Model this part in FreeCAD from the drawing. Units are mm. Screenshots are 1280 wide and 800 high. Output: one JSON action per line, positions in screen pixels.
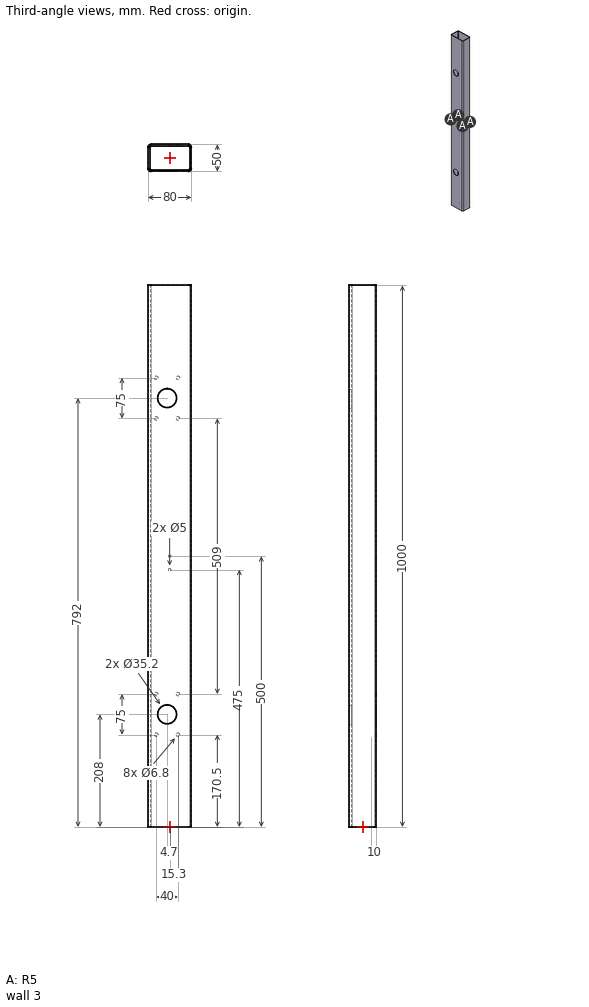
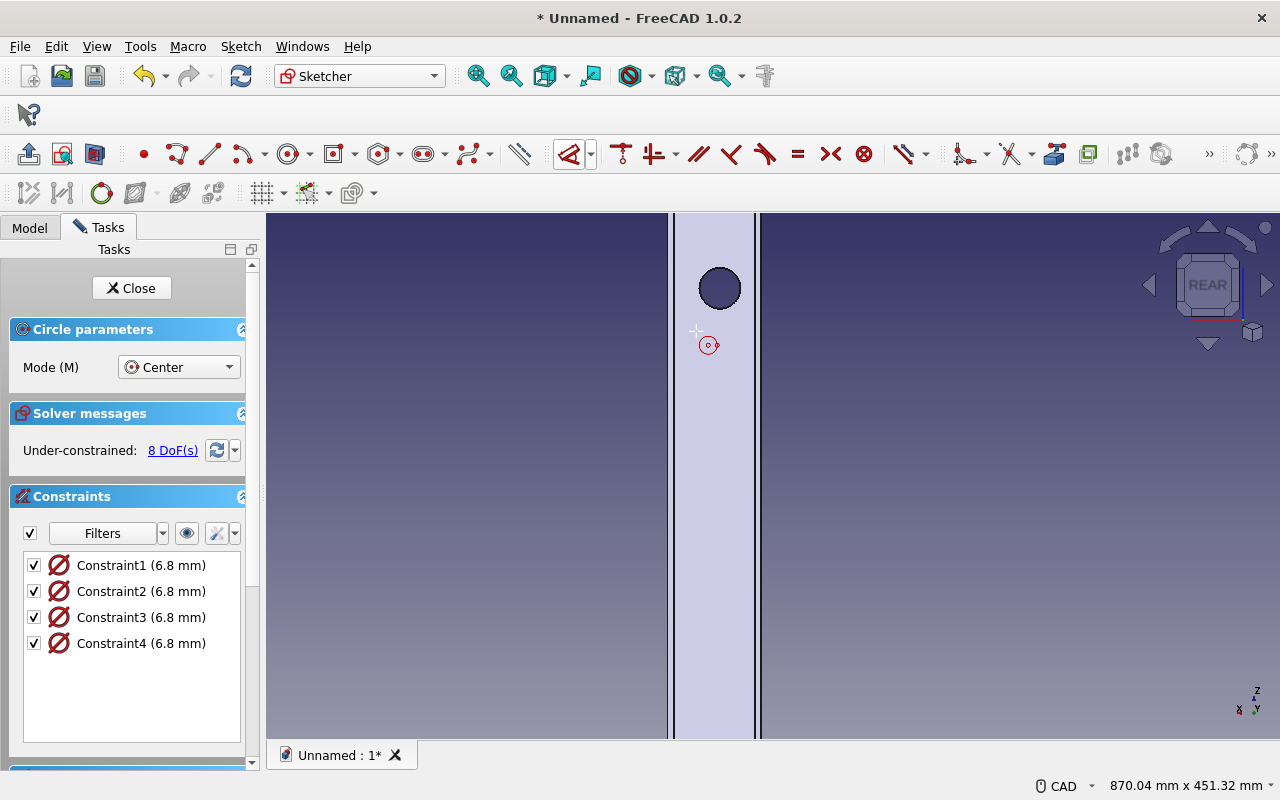
{"action": "left_click", "coordinate": [697, 332]}
{"action": "mouse_move", "coordinate": [699, 329]}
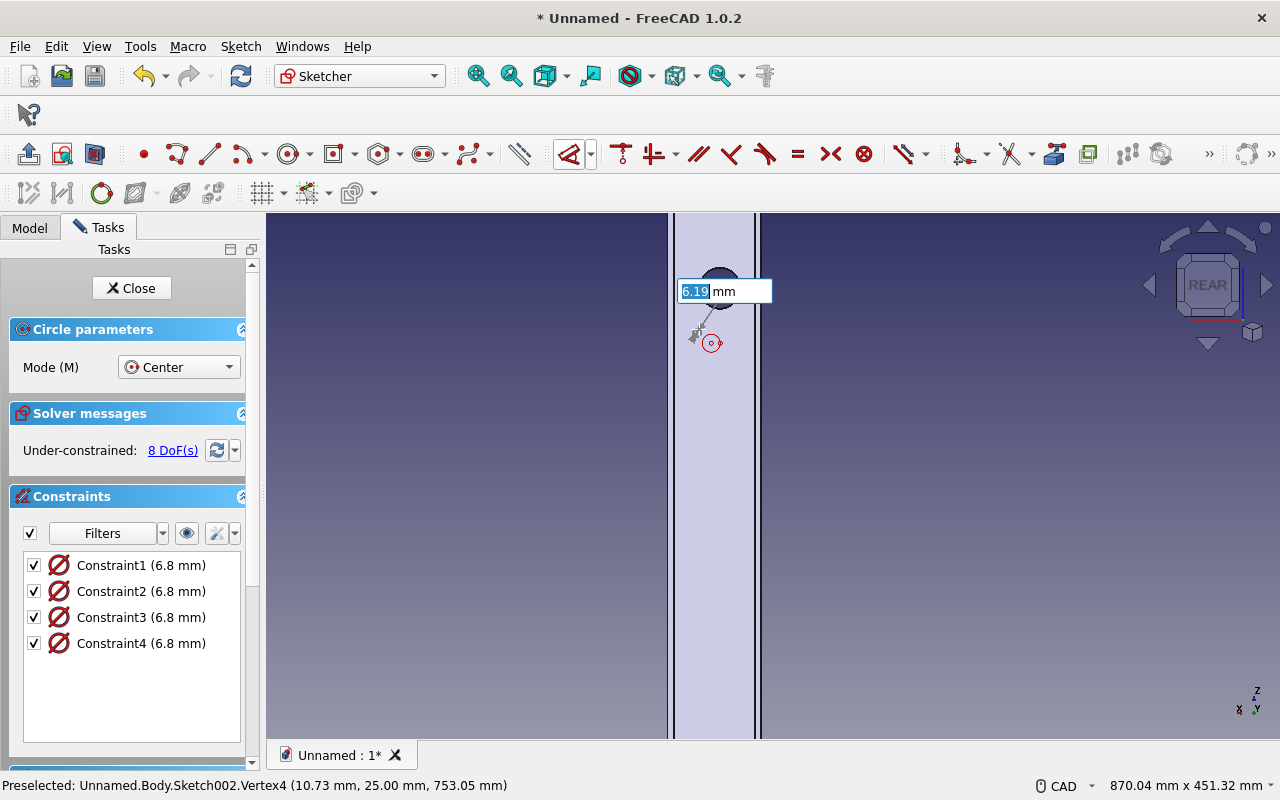
{"action": "type", "text": "6.8"}
{"action": "key", "text": "Return"}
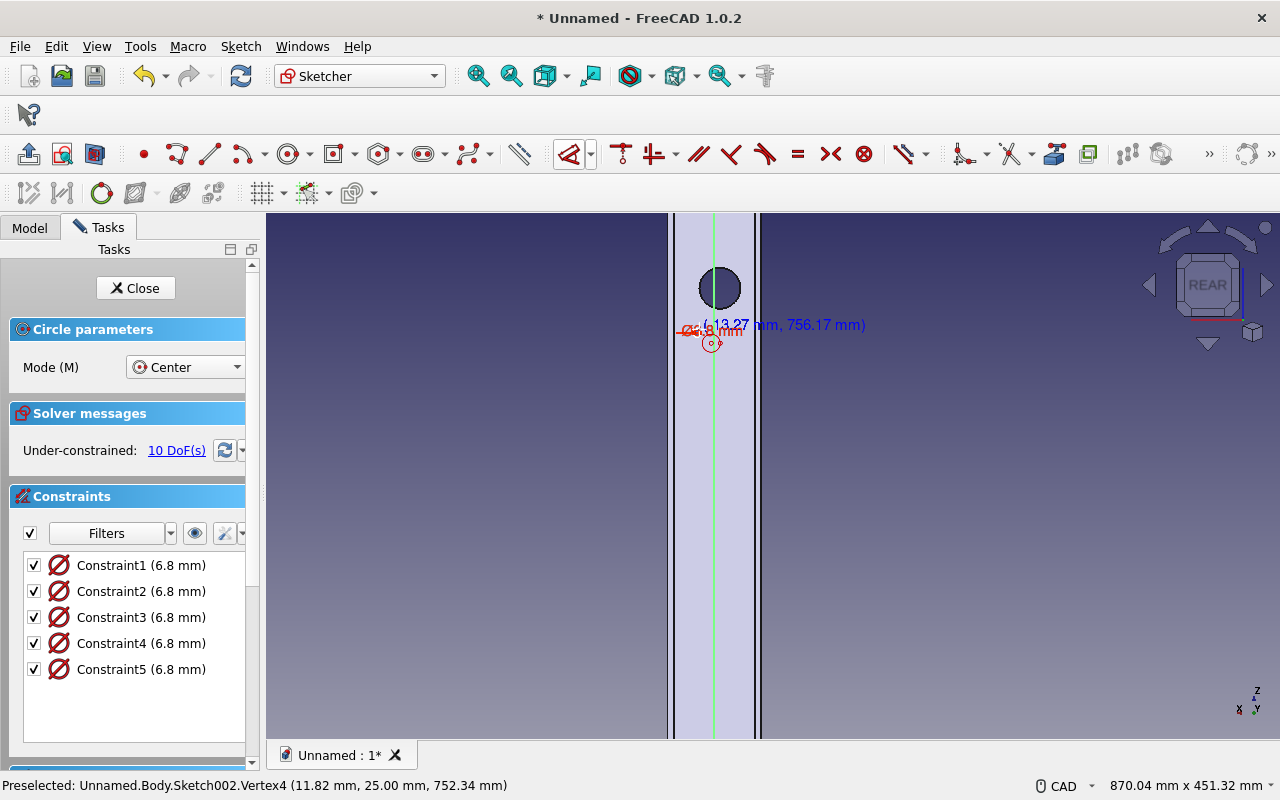
{"action": "scroll", "coordinate": [743, 332], "scroll_direction": "up", "scroll_amount": 9}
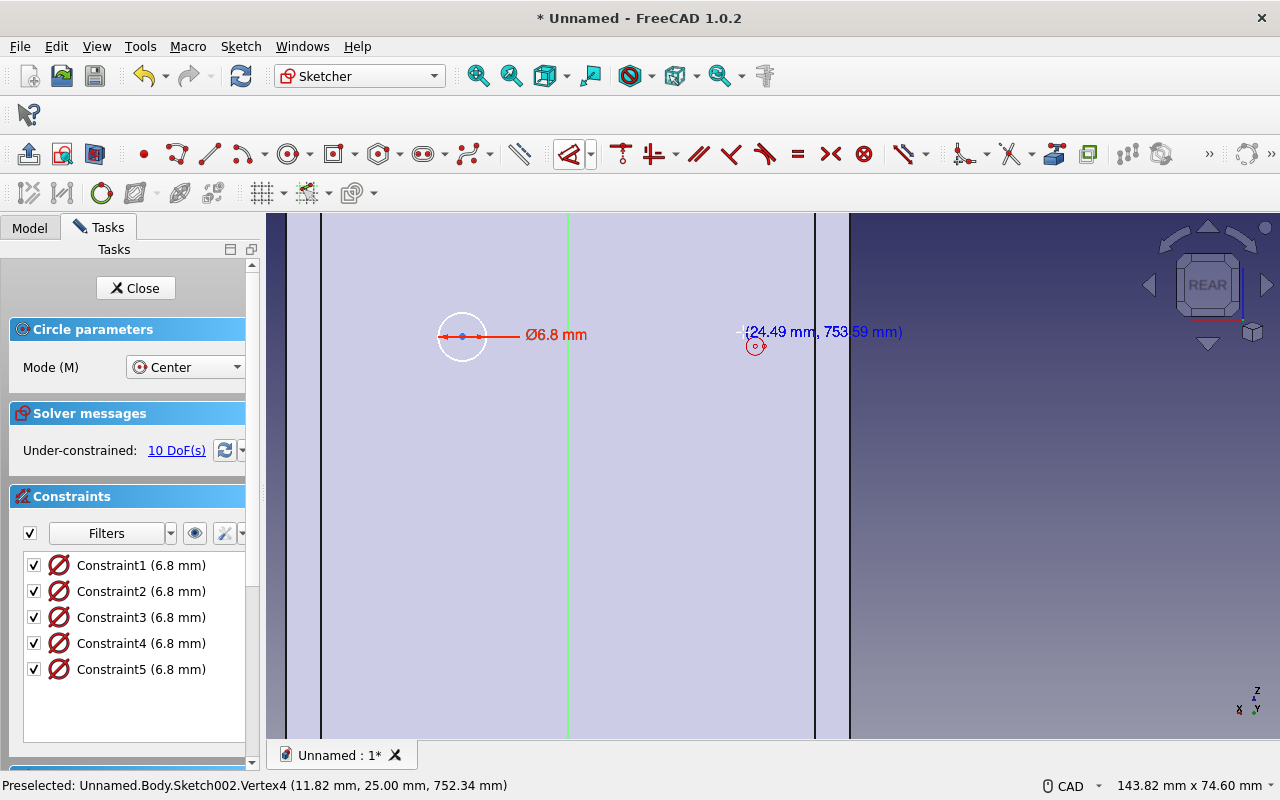
{"action": "scroll", "coordinate": [711, 331], "scroll_direction": "down", "scroll_amount": 14}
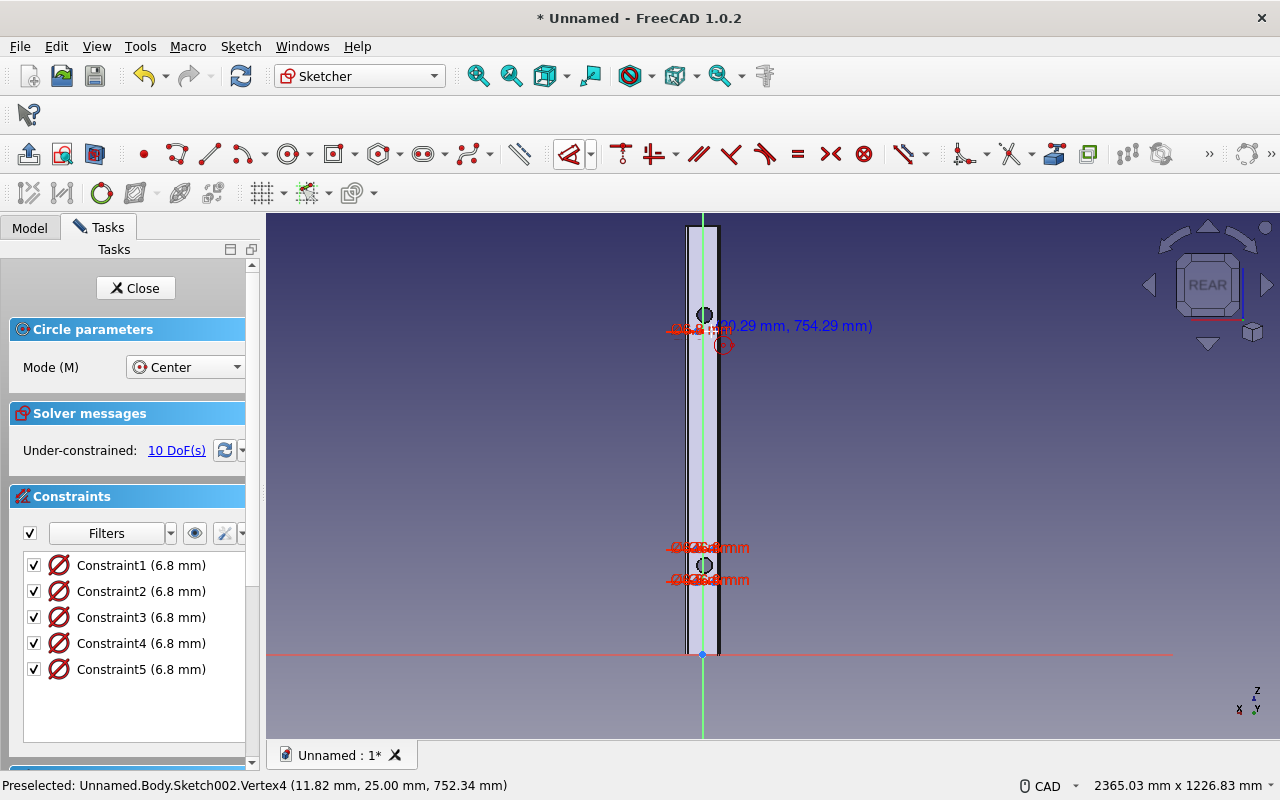
{"action": "scroll", "coordinate": [713, 331], "scroll_direction": "up", "scroll_amount": 3}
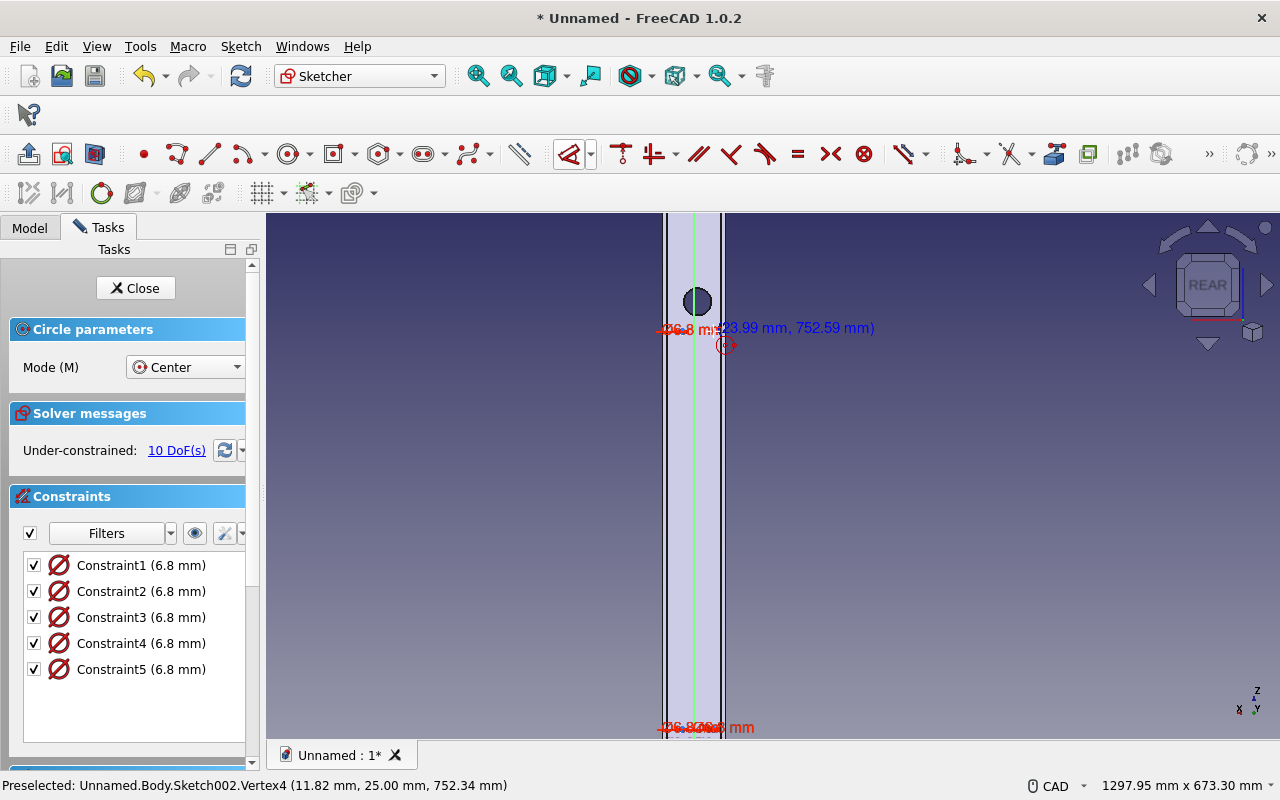
{"action": "left_click", "coordinate": [713, 331]}
{"action": "mouse_move", "coordinate": [715, 329]}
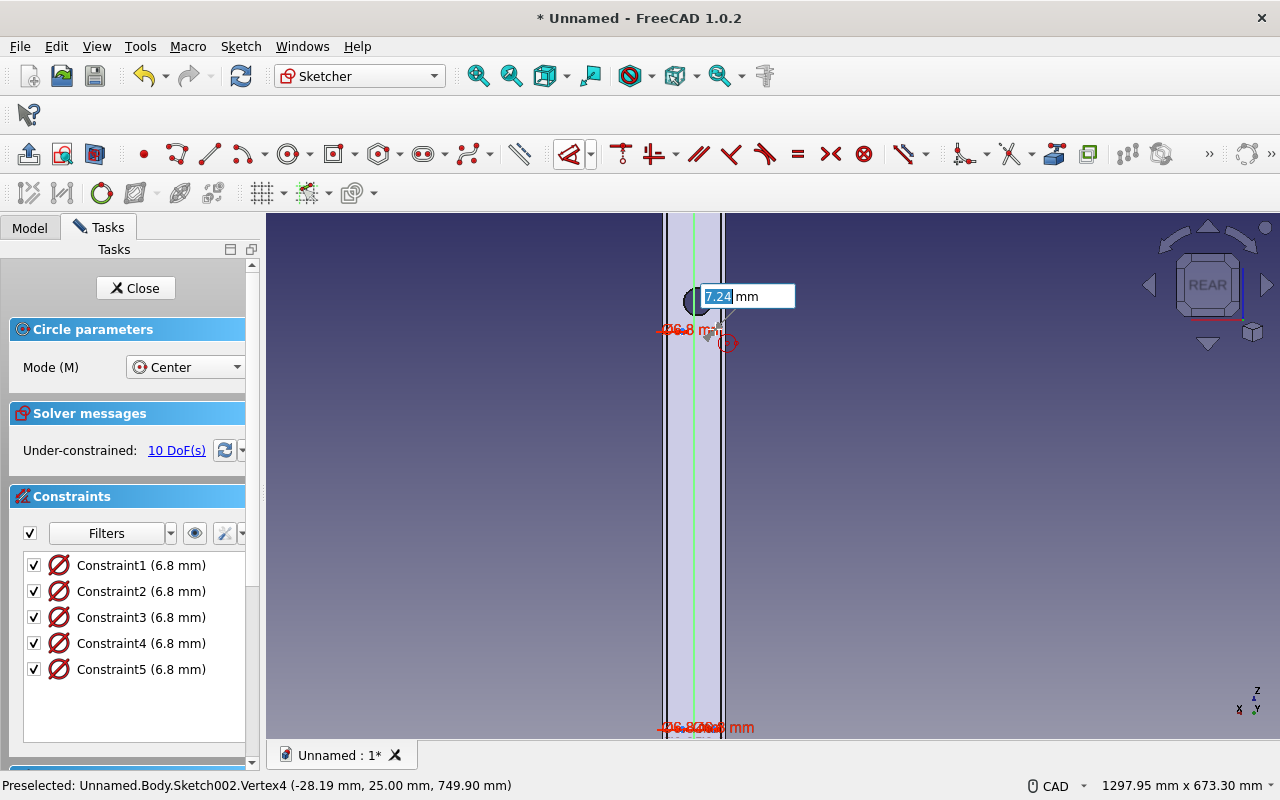
{"action": "type", "text": "6.8"}
{"action": "key", "text": "Return"}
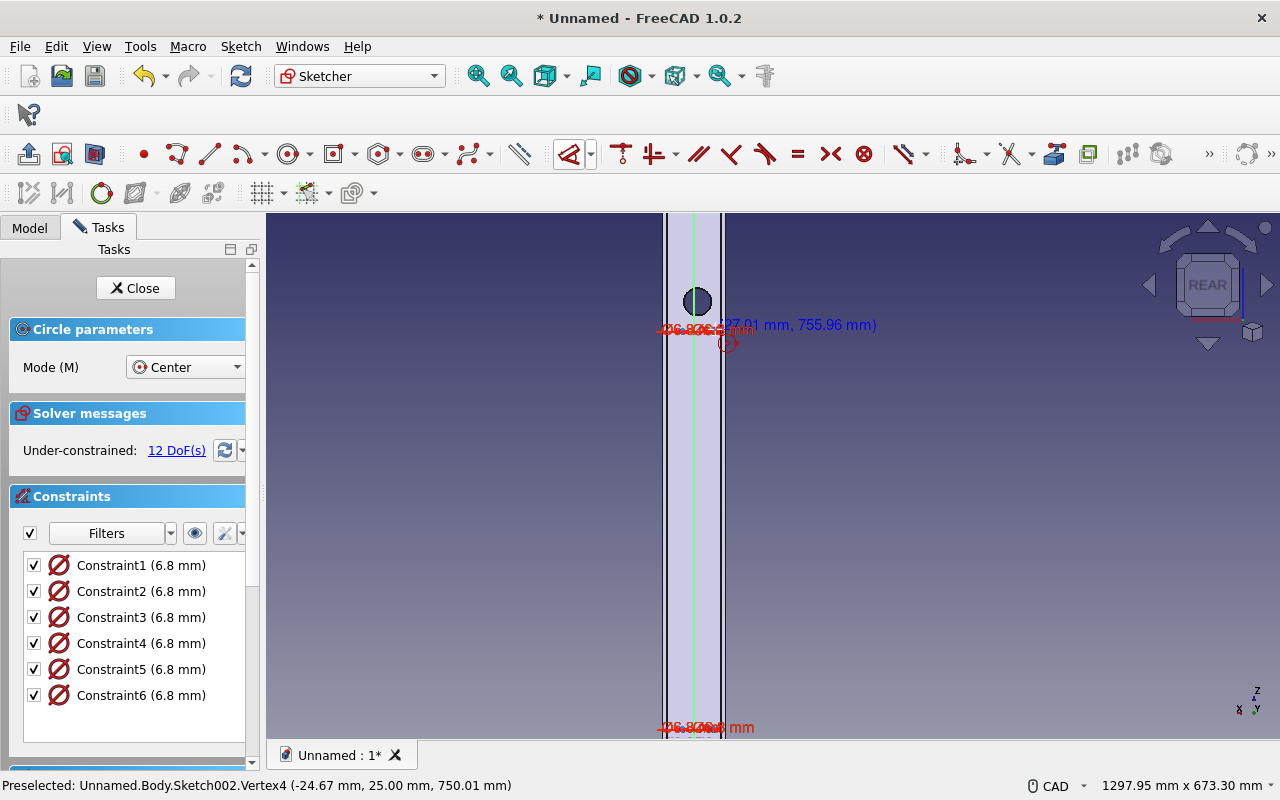
{"action": "scroll", "coordinate": [713, 273], "scroll_direction": "up", "scroll_amount": 11}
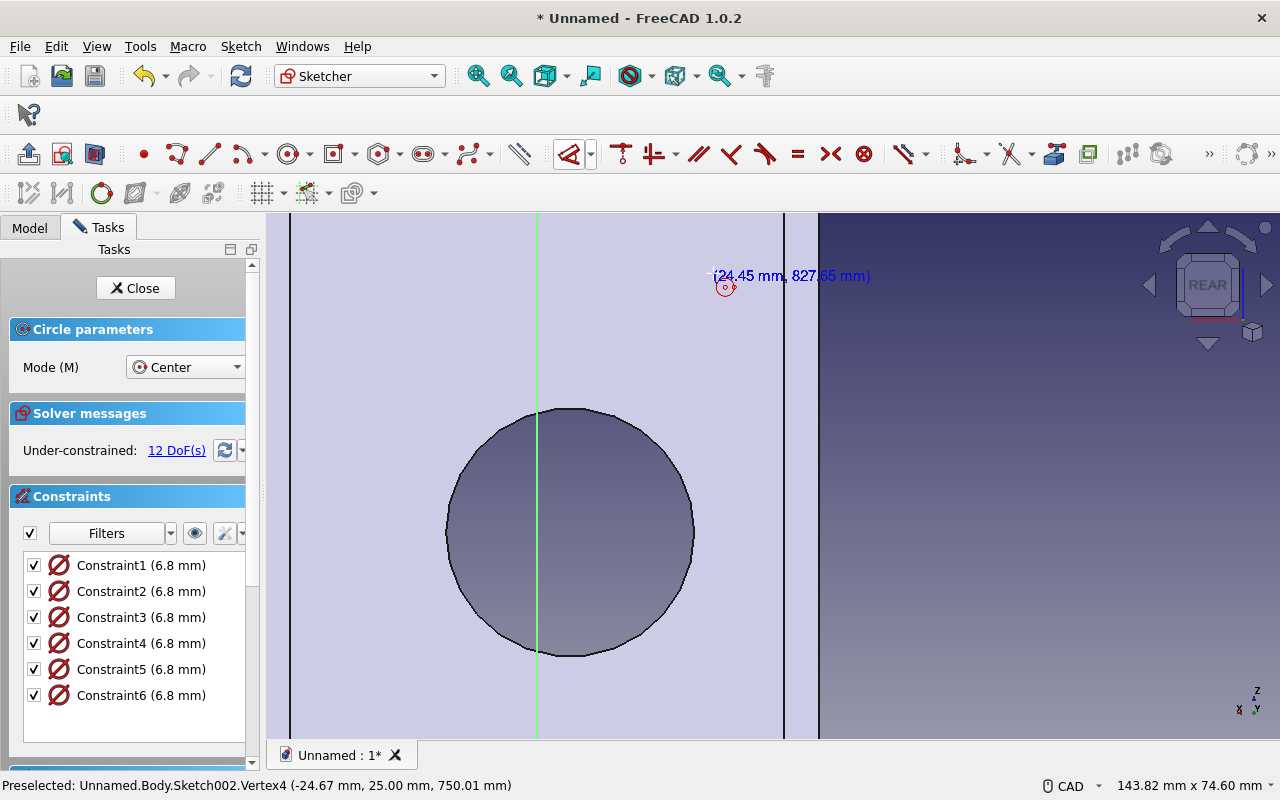
{"action": "scroll", "coordinate": [713, 301], "scroll_direction": "down", "scroll_amount": 14}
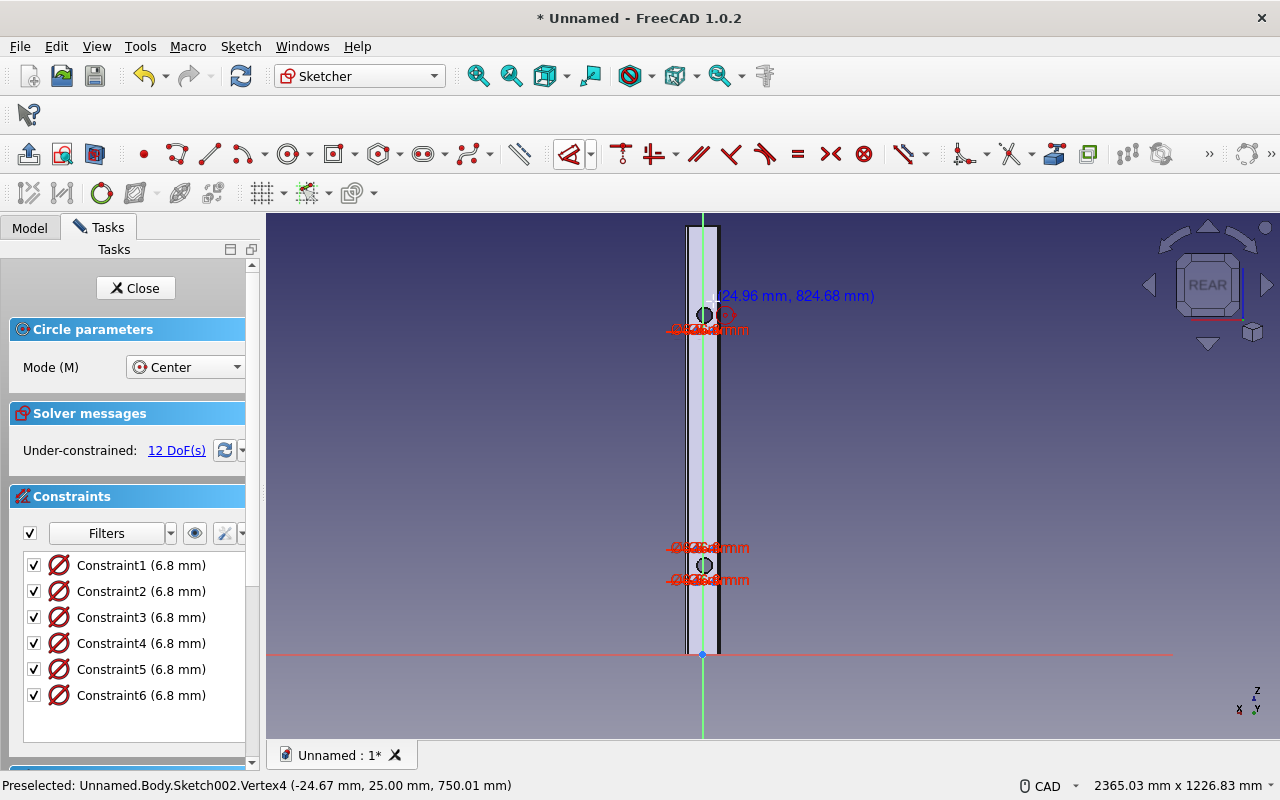
{"action": "scroll", "coordinate": [713, 299], "scroll_direction": "up", "scroll_amount": 3}